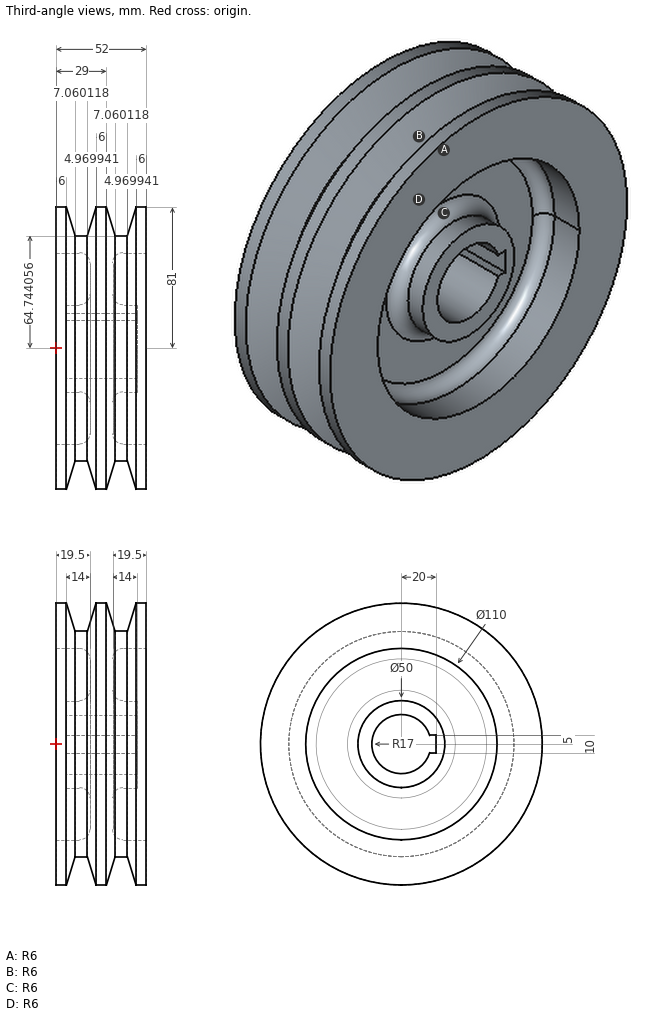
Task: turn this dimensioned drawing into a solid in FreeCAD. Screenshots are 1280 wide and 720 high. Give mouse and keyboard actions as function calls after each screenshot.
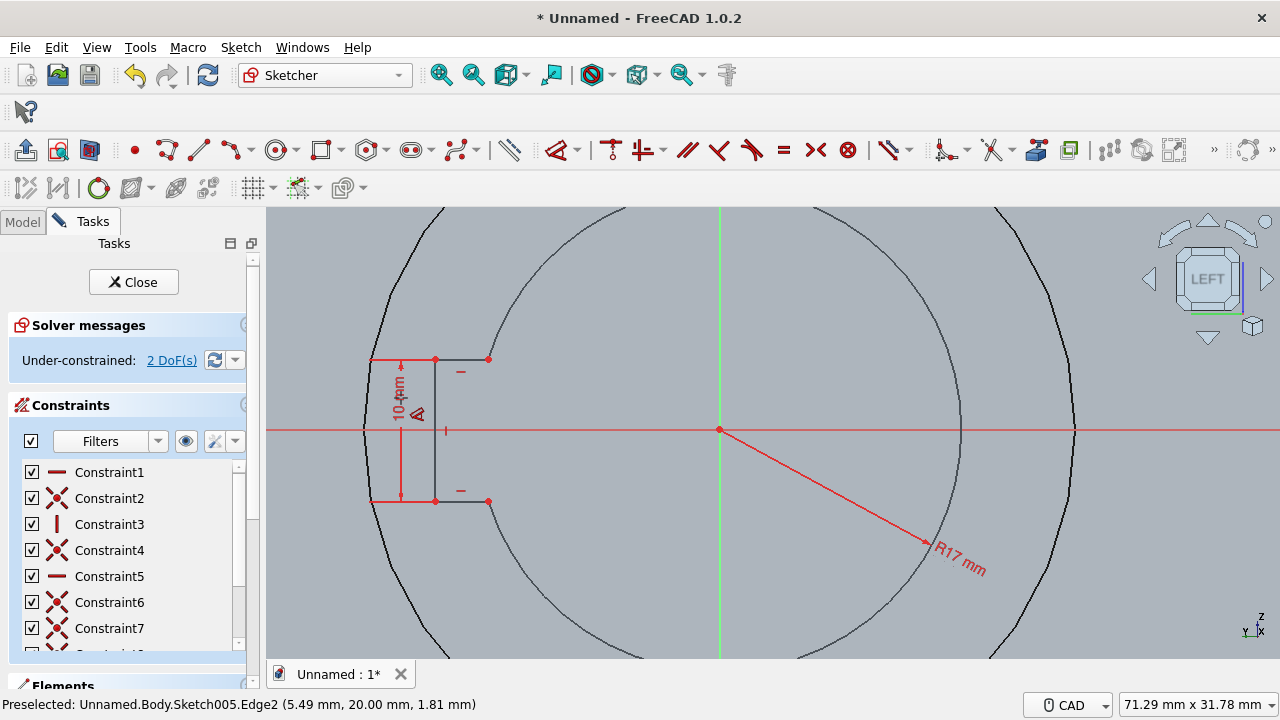
click(488, 360)
click(754, 395)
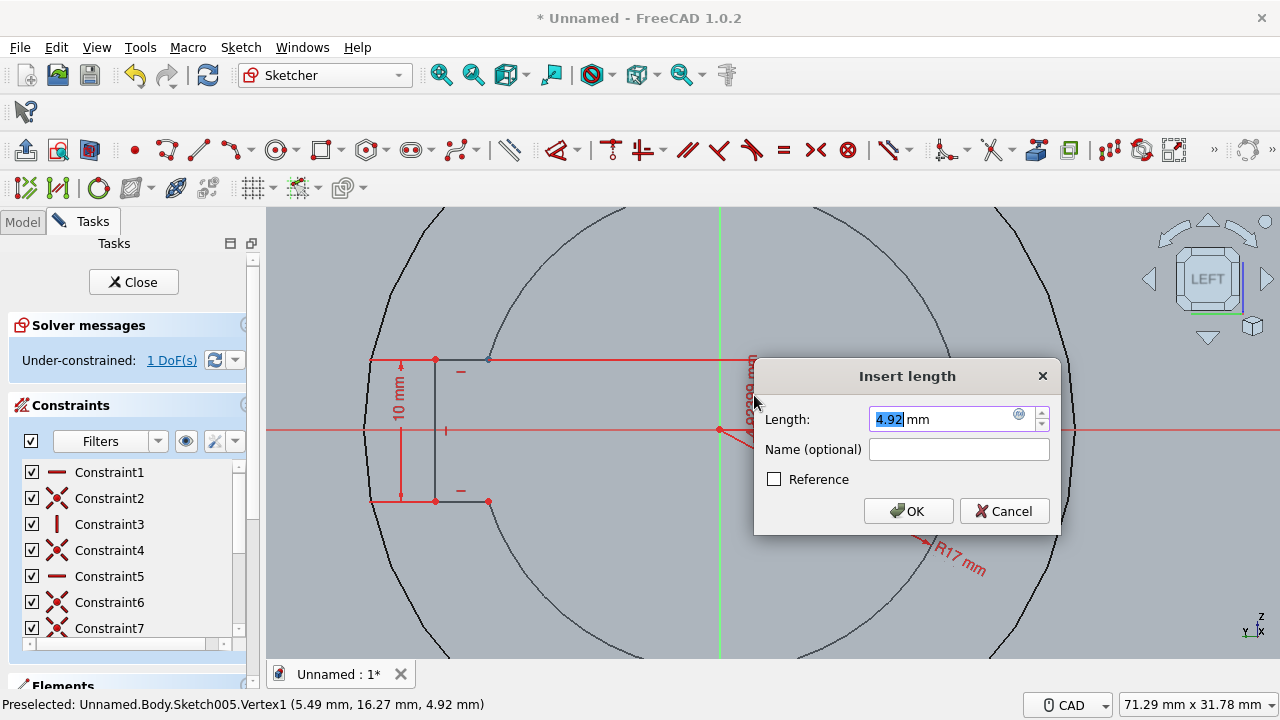
text(5)
key(Return)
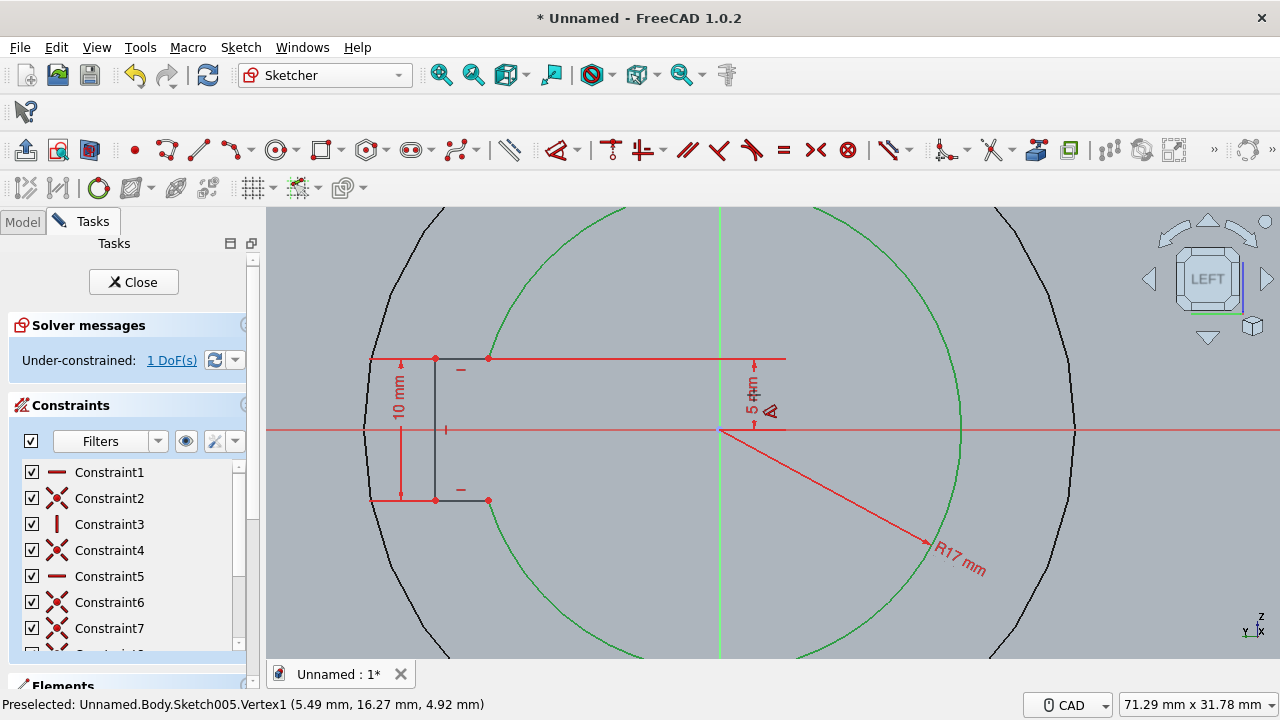
click(435, 359)
click(577, 325)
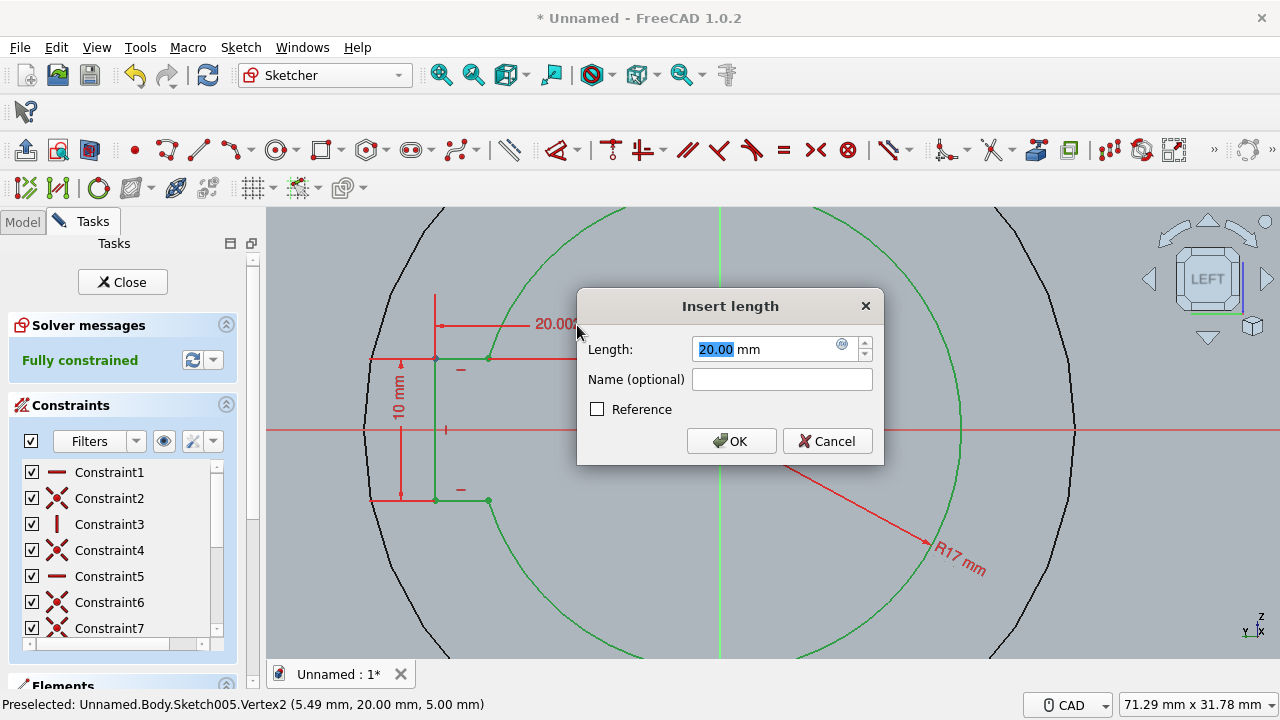
text(20)
key(Return)
key(Escape)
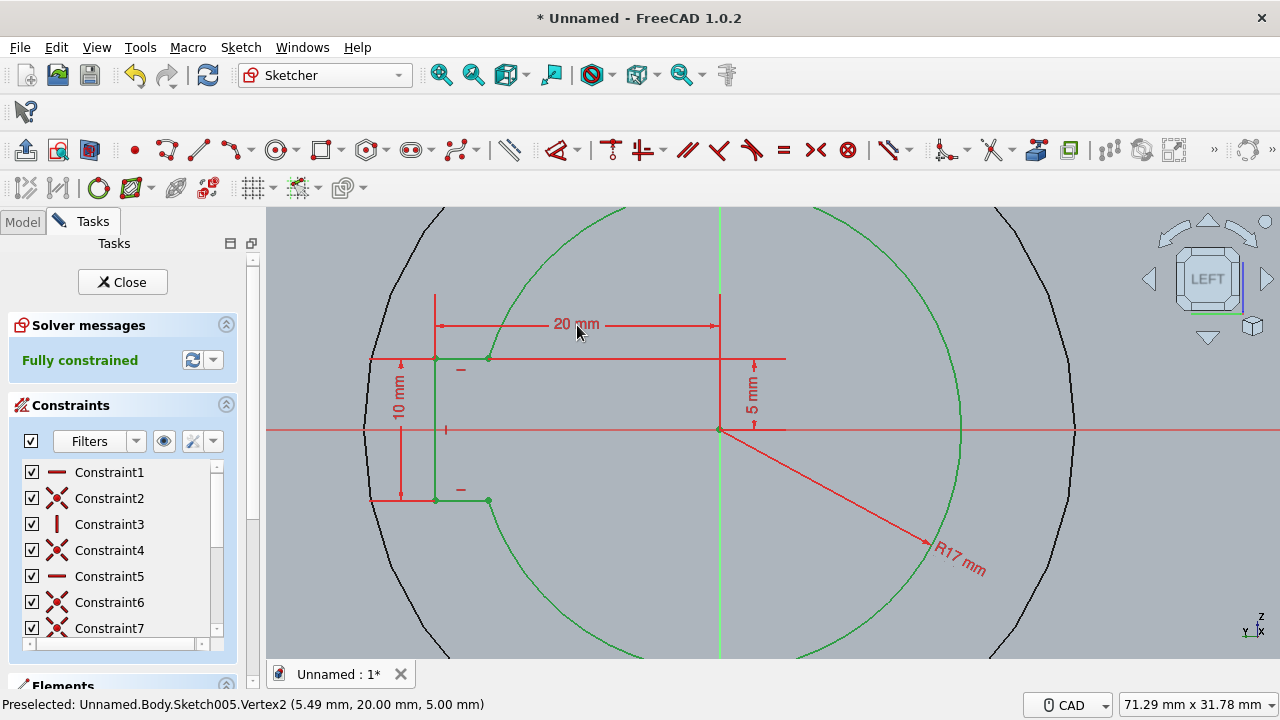
click(123, 282)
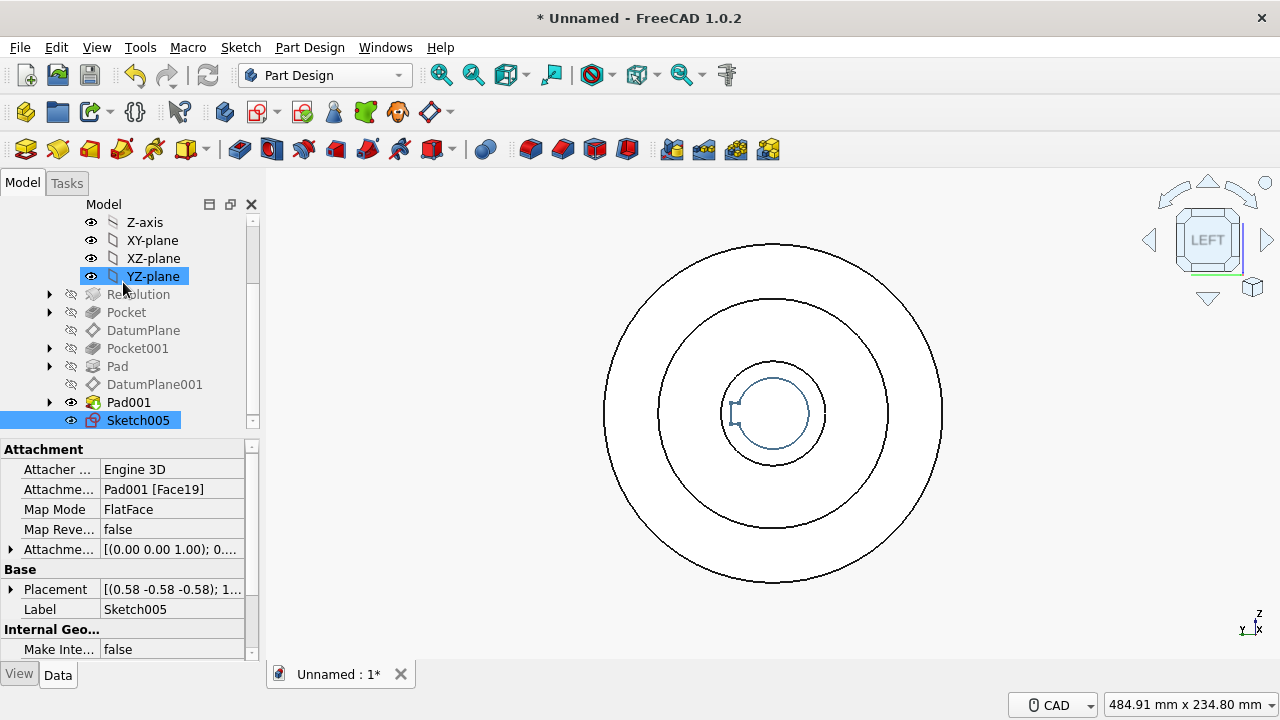
click(240, 150)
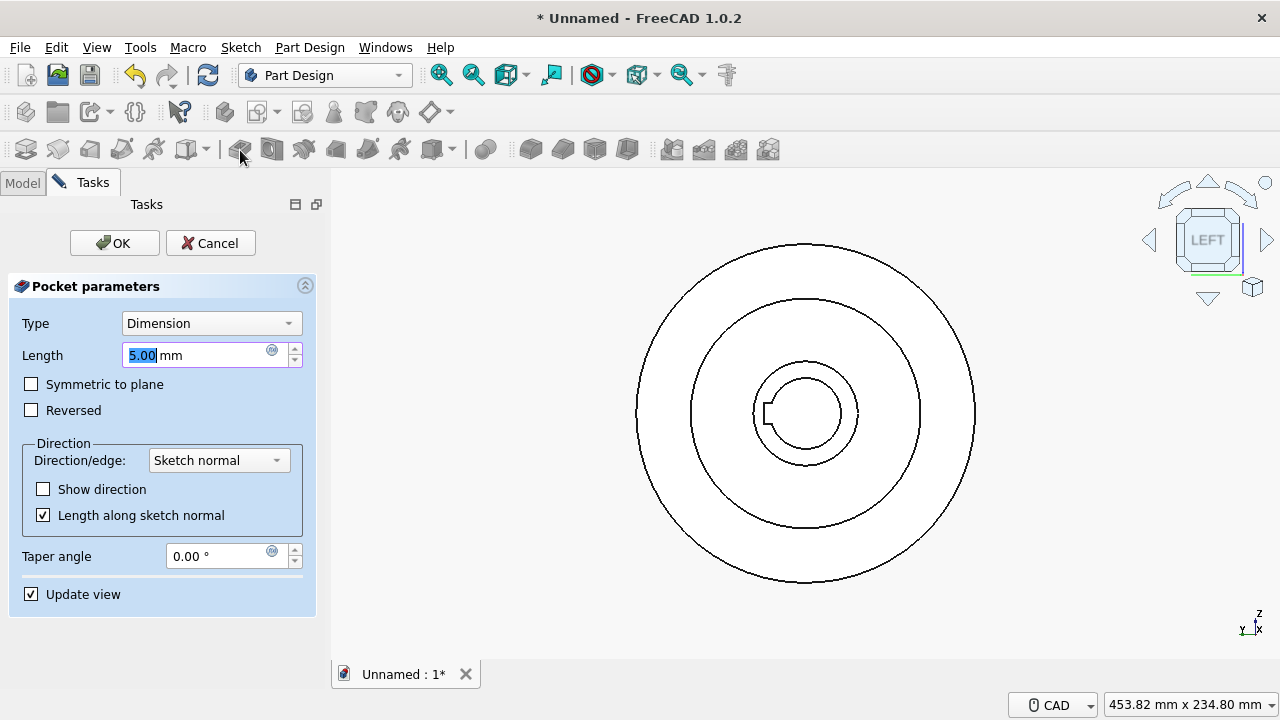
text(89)
key(Tab)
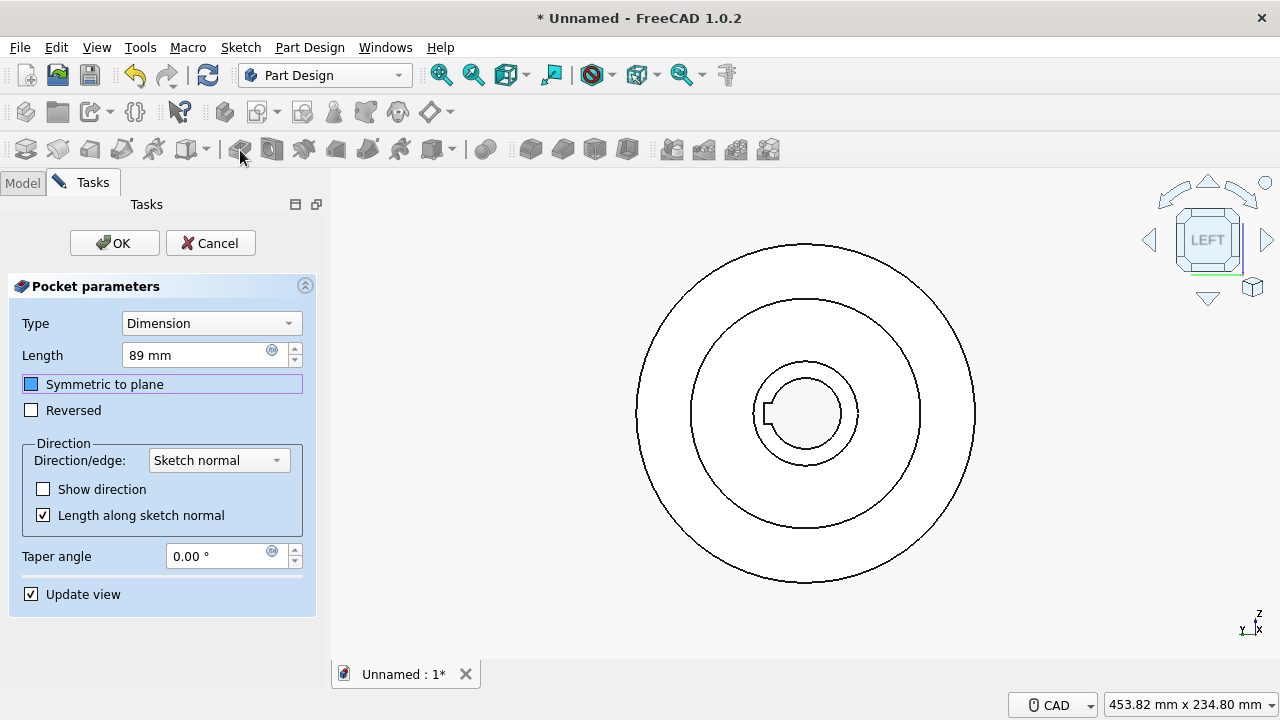
click(115, 243)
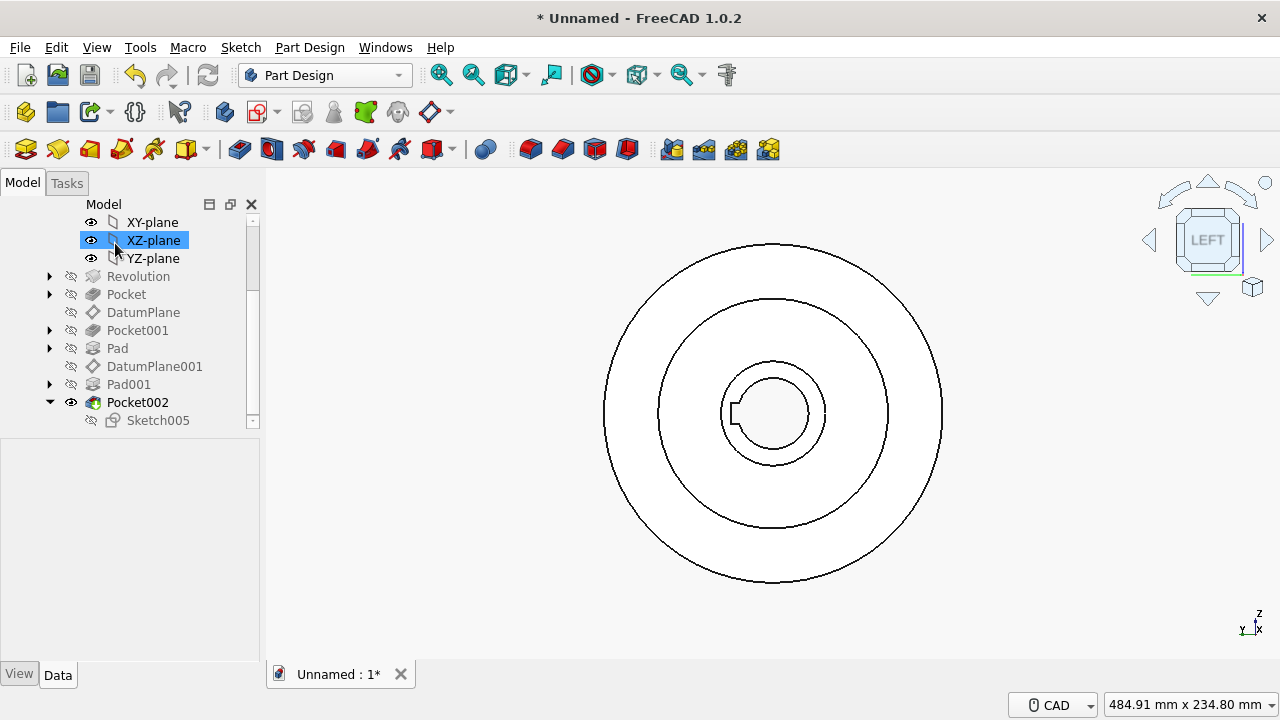
key(0)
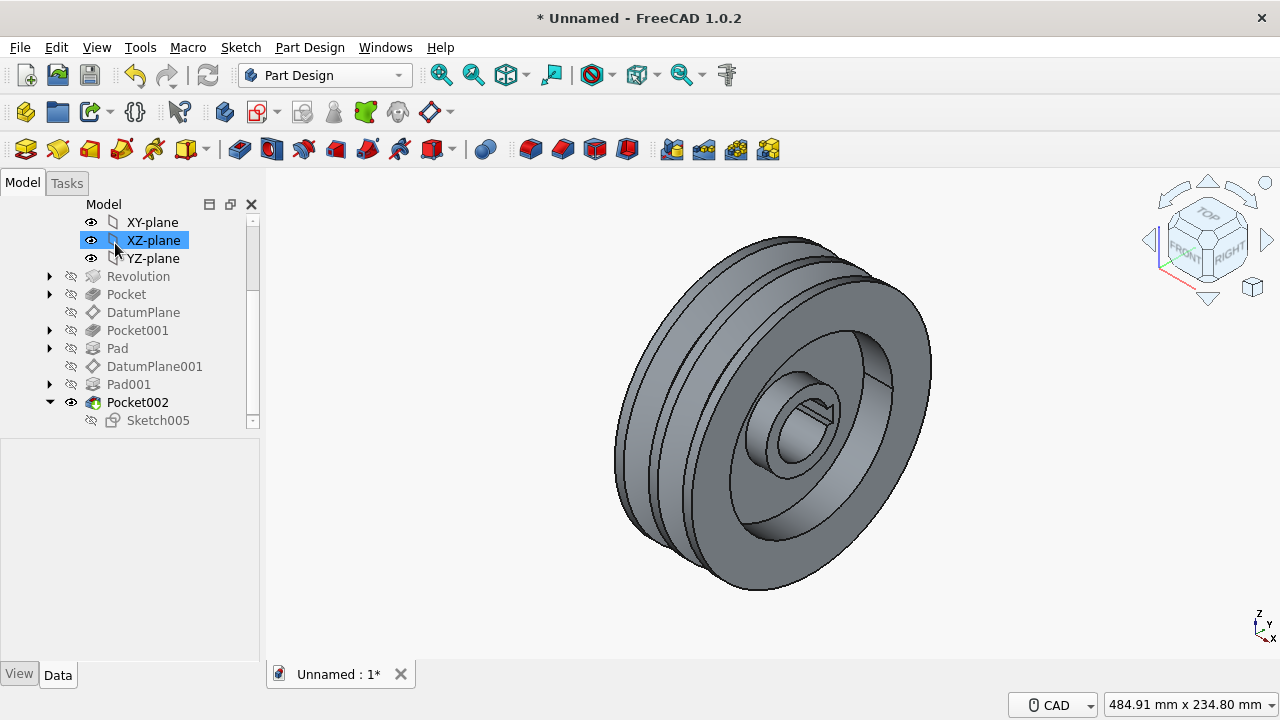
key(2)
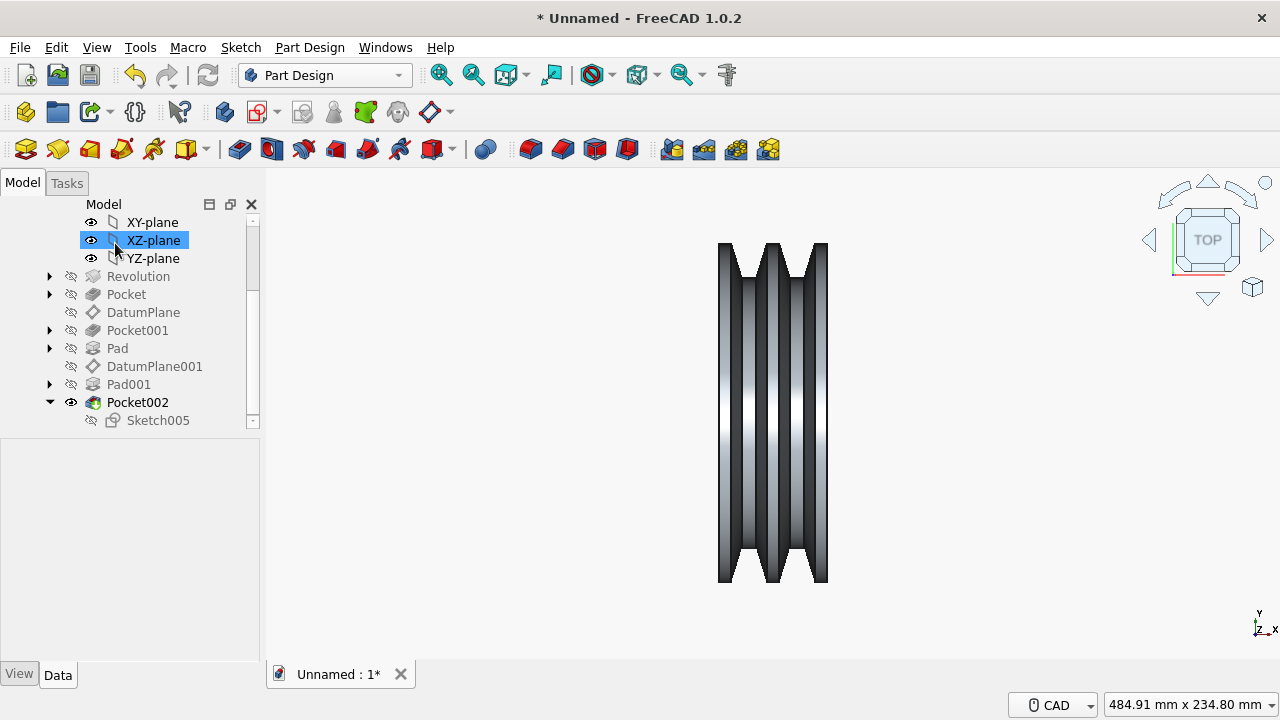
key(1)